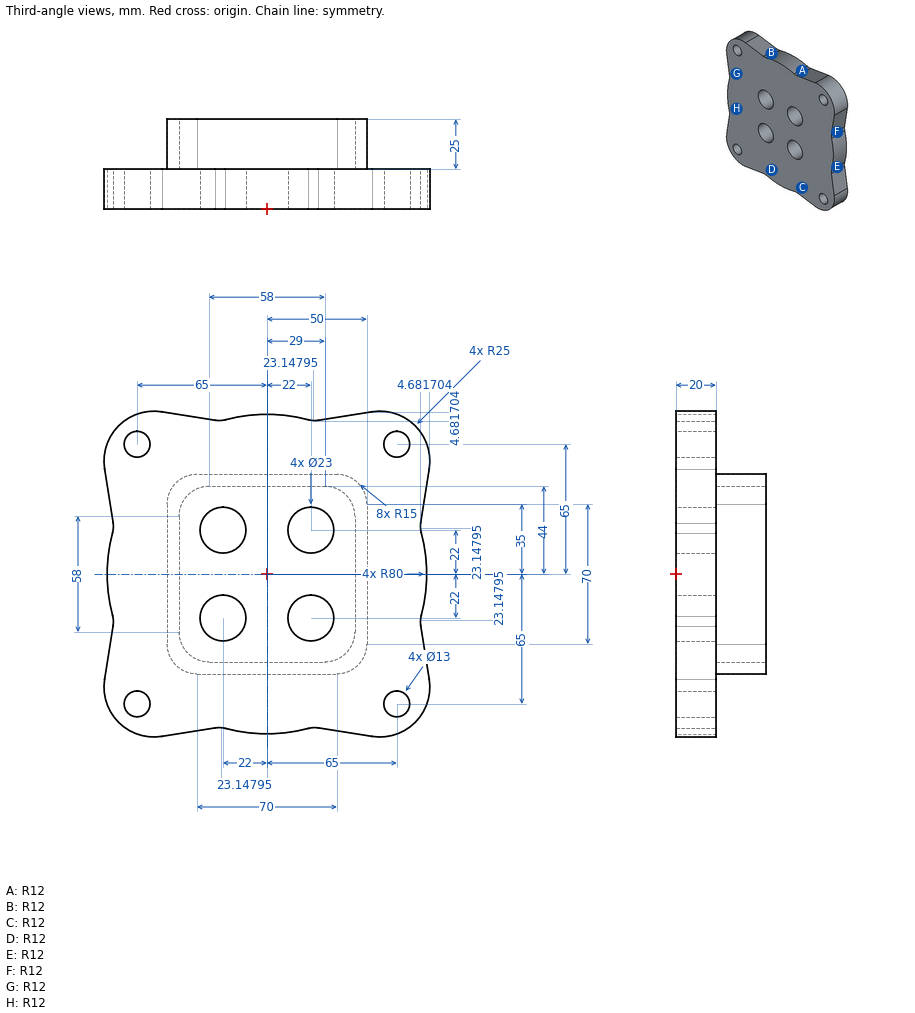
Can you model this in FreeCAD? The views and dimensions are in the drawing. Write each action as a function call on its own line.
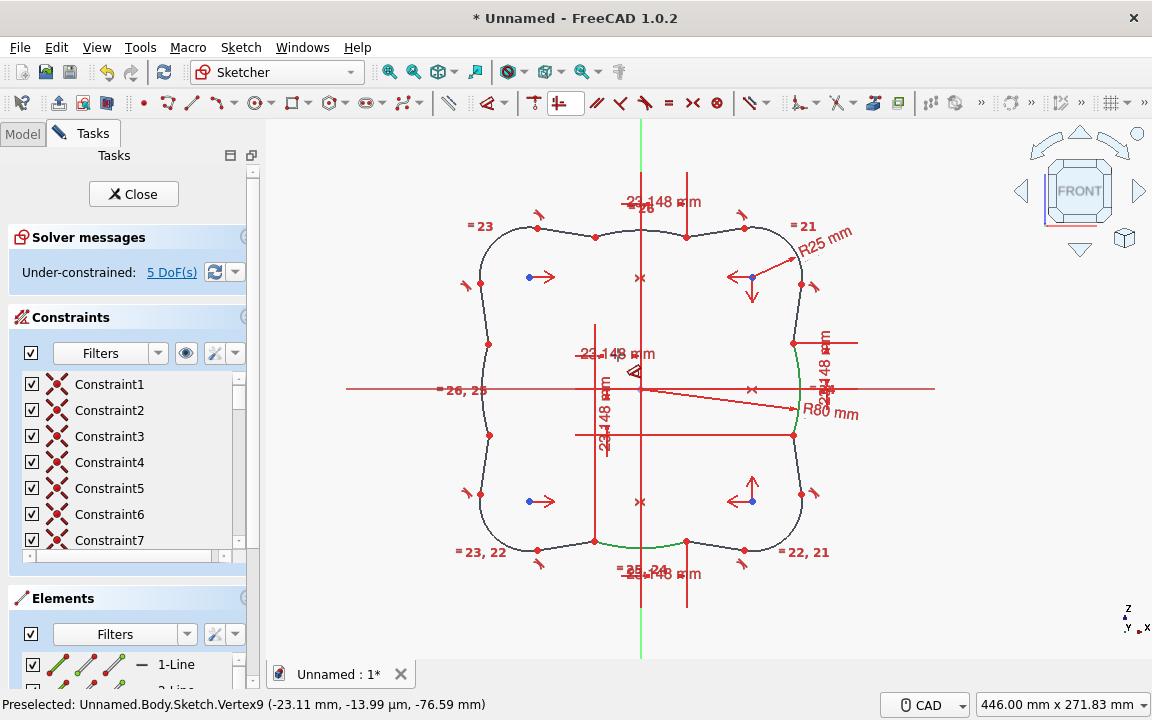
click(489, 436)
click(455, 413)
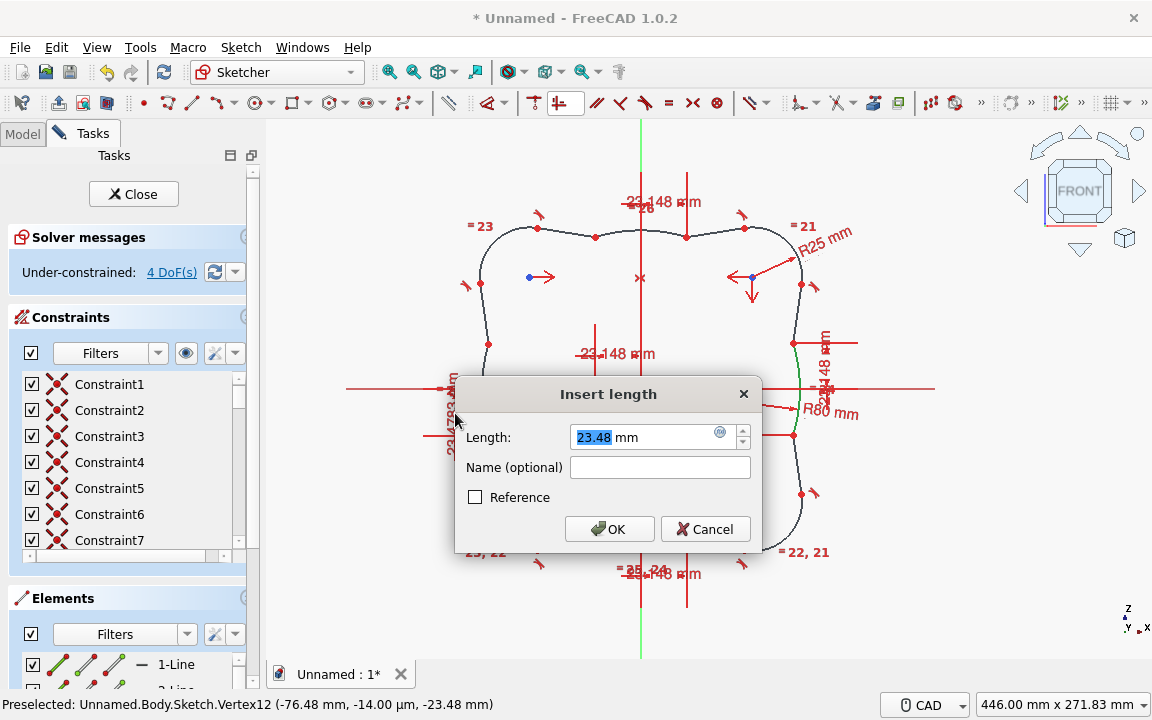
text(23.14795)
key(Return)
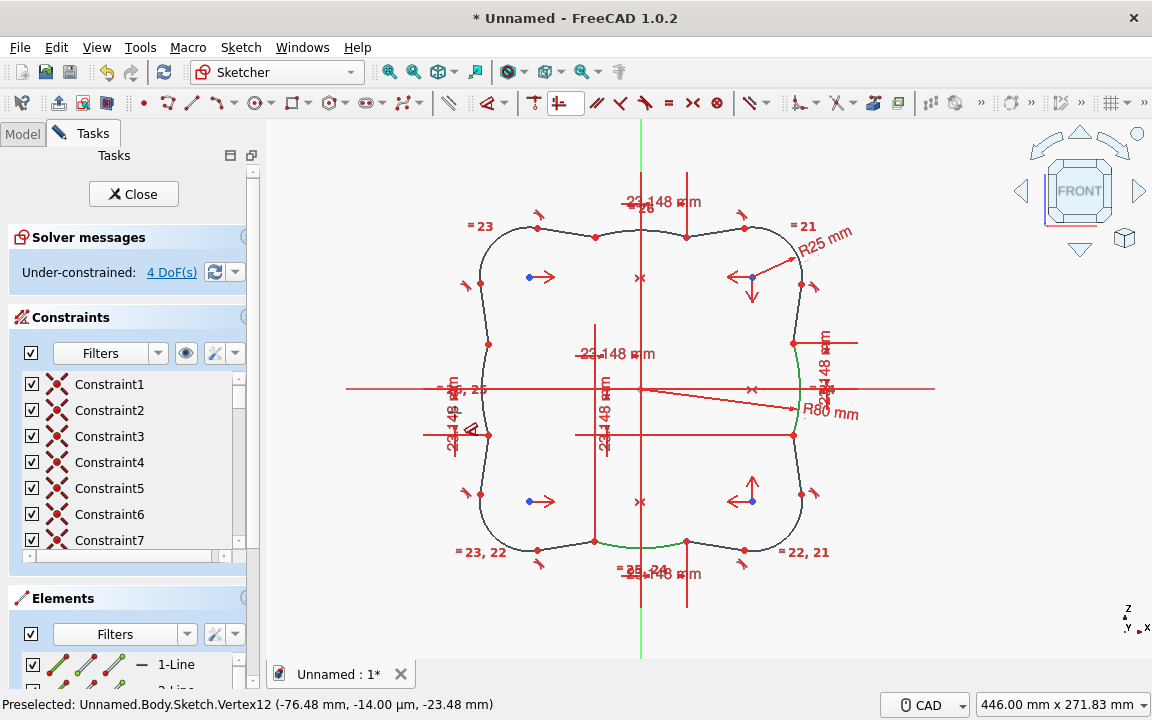
click(489, 344)
click(455, 367)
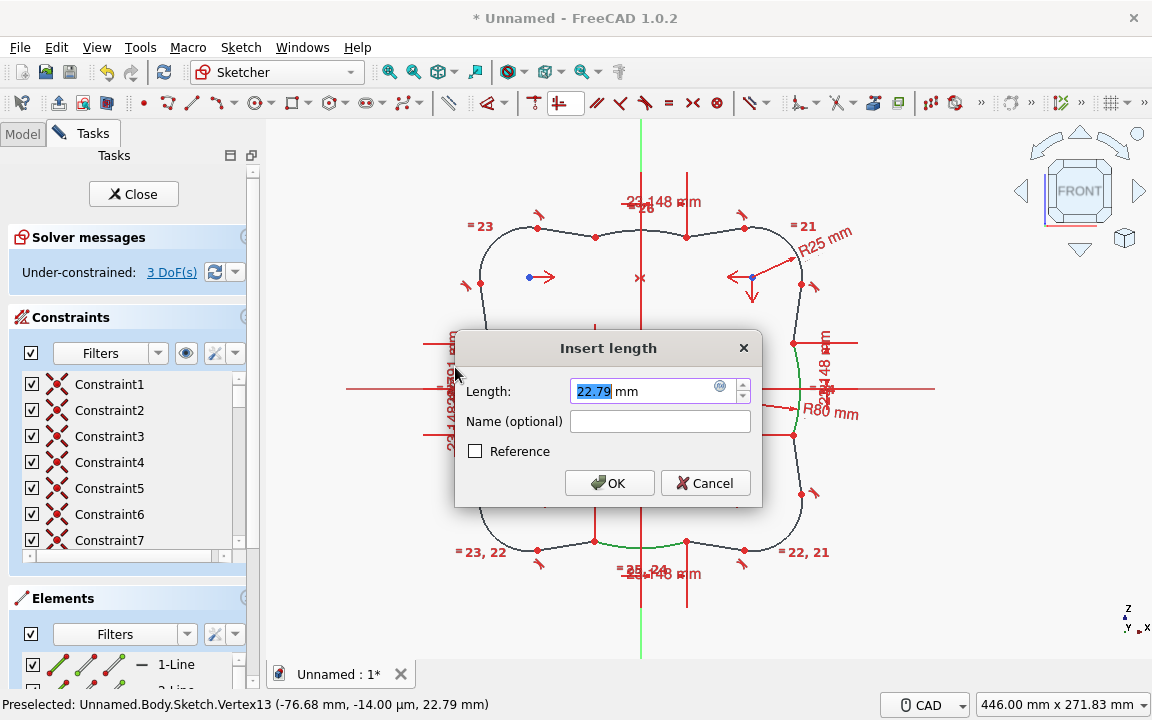
text(23.14795)
key(Return)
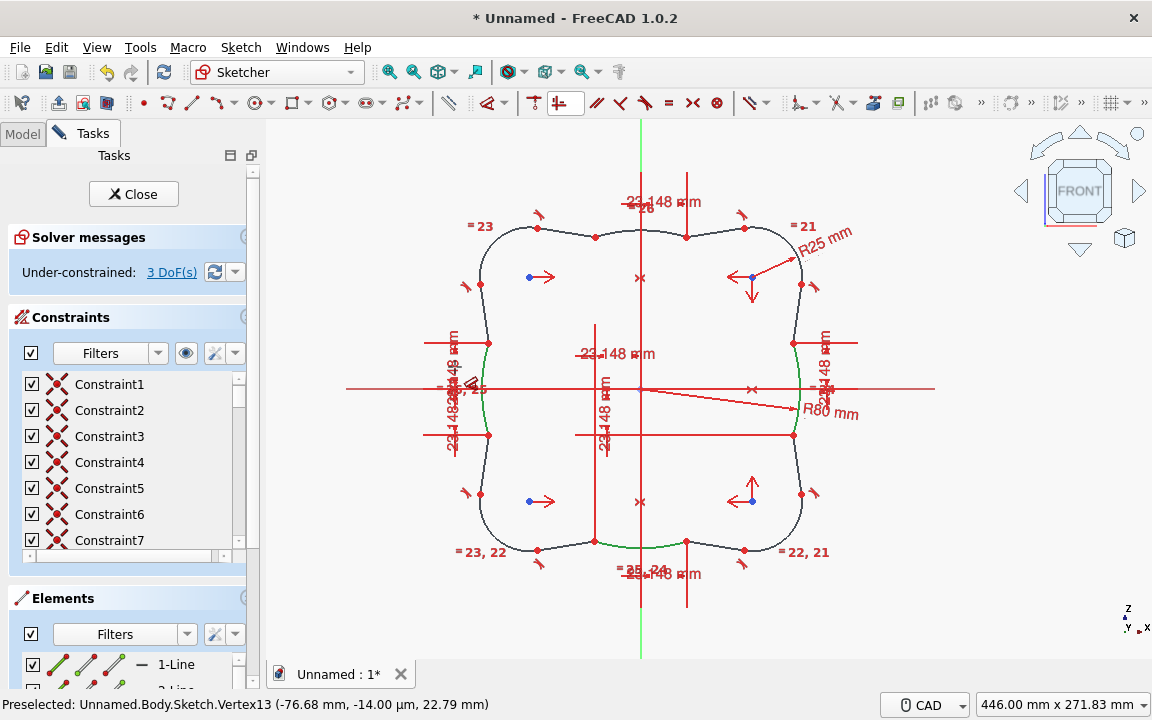
click(595, 237)
click(618, 179)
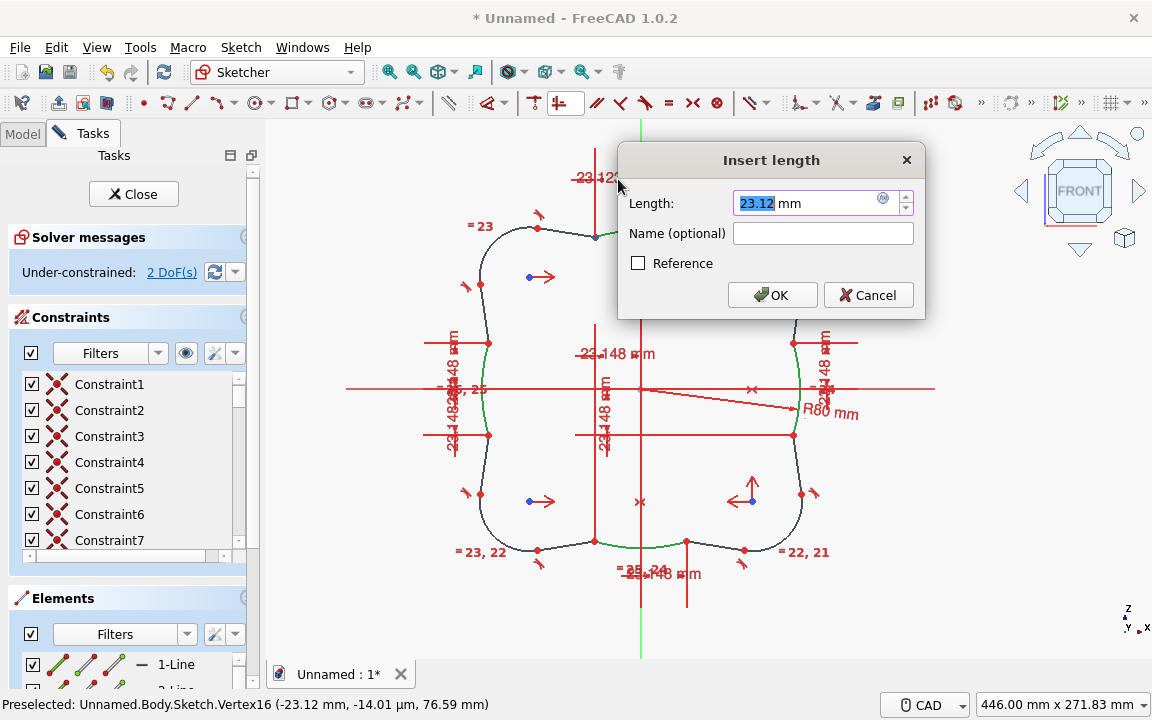
text(23.14795)
key(Return)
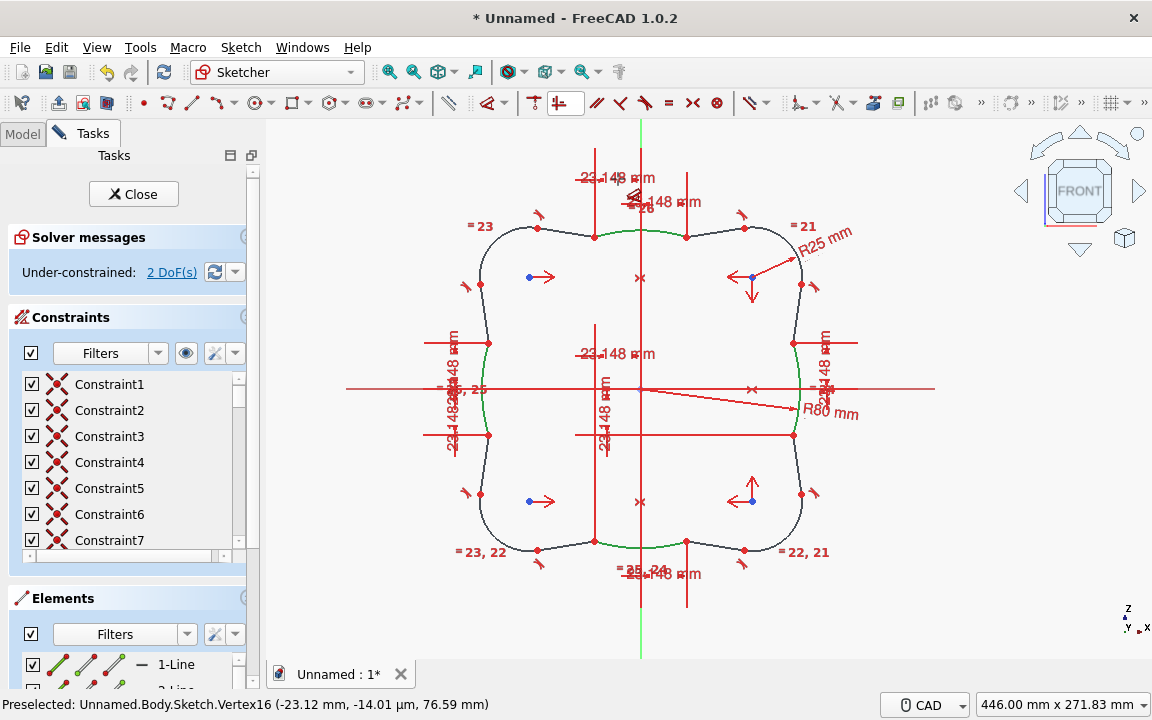
scroll(704, 234, up, 8)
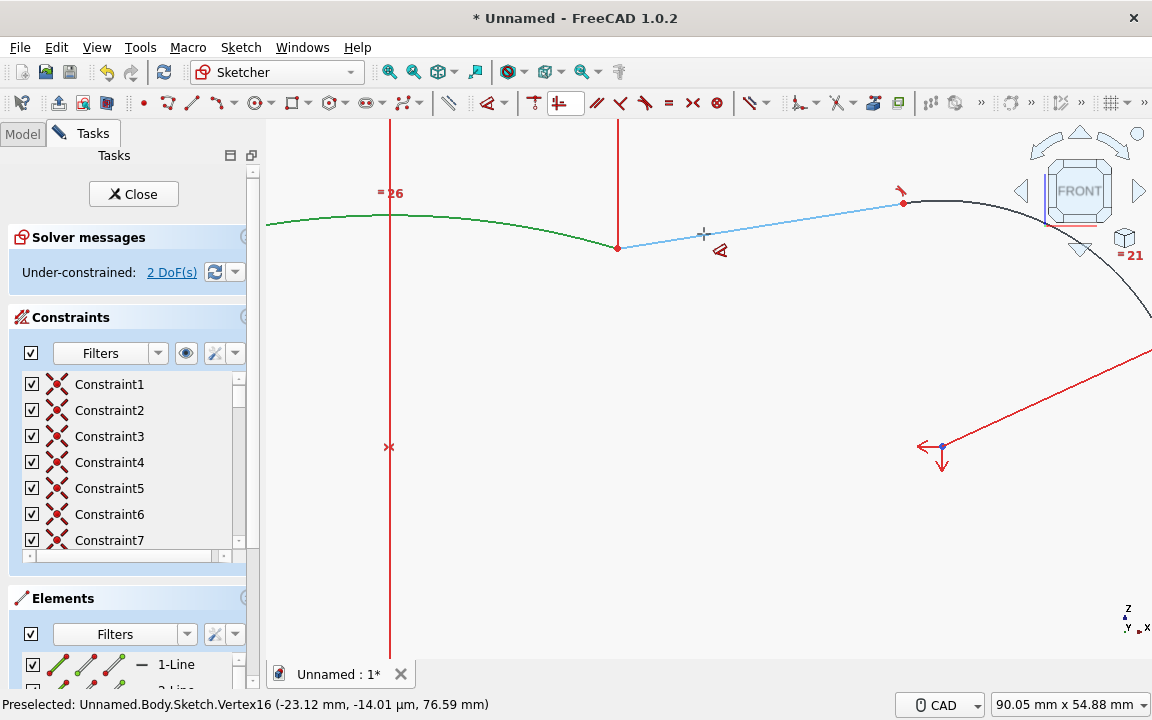
click(703, 235)
click(937, 226)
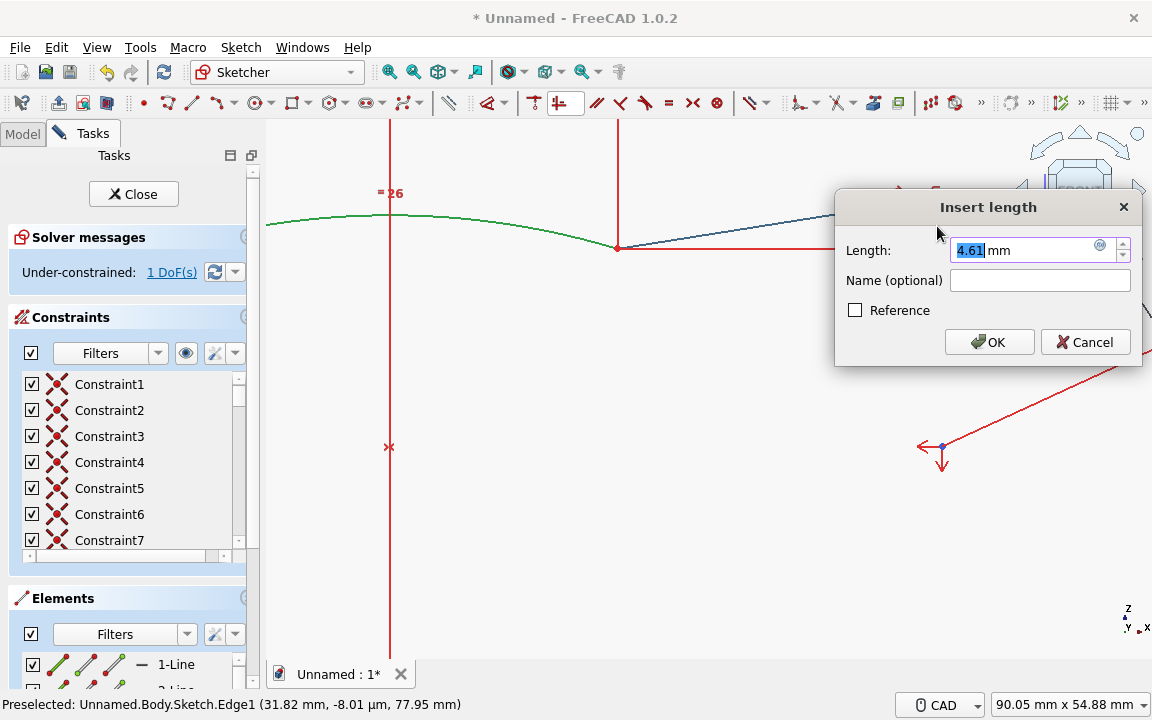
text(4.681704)
key(Return)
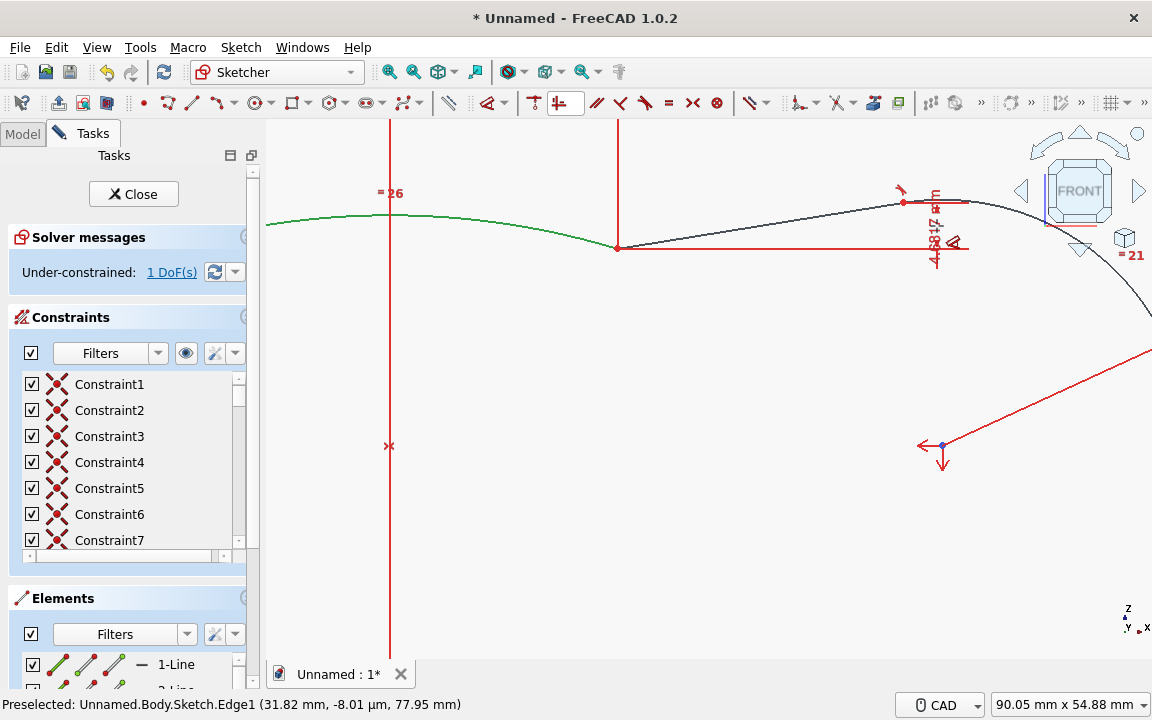
scroll(704, 234, down, 8)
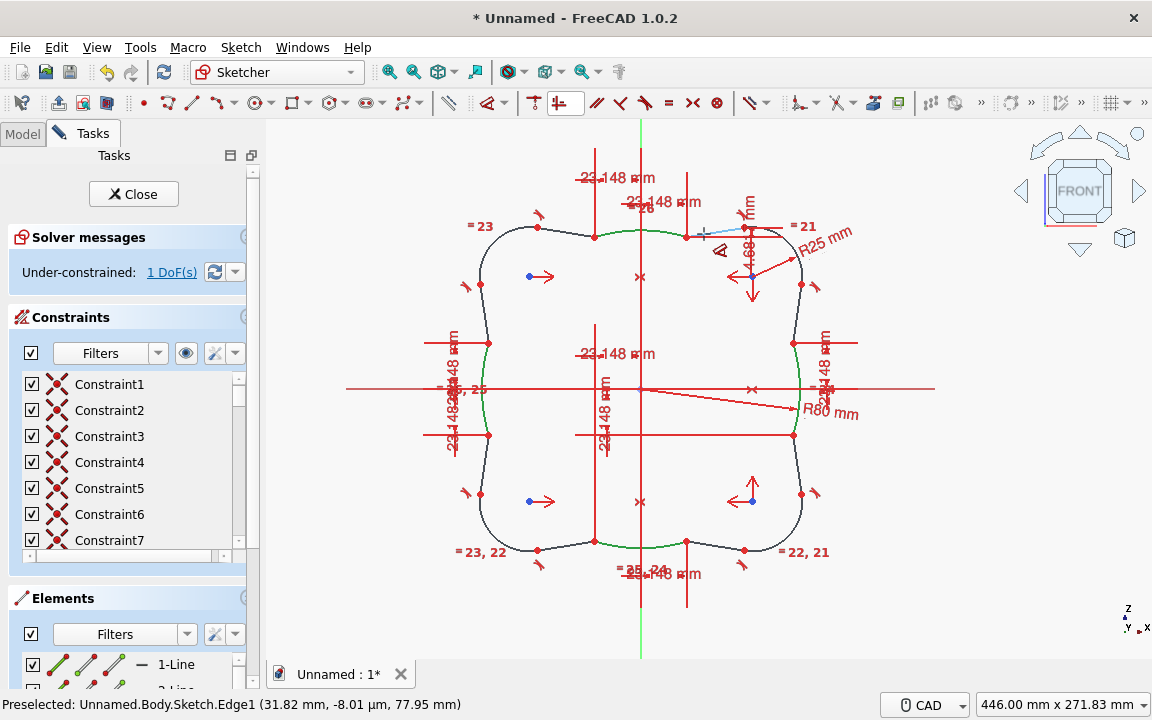
scroll(799, 302, up, 8)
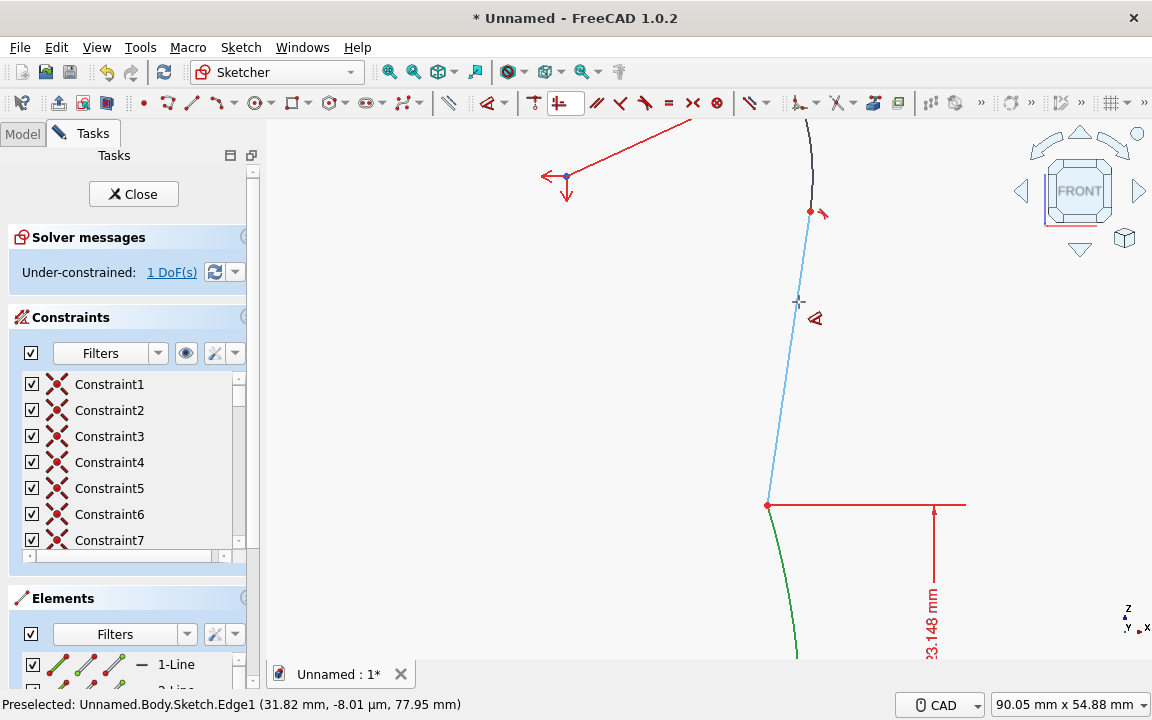
click(797, 300)
click(789, 178)